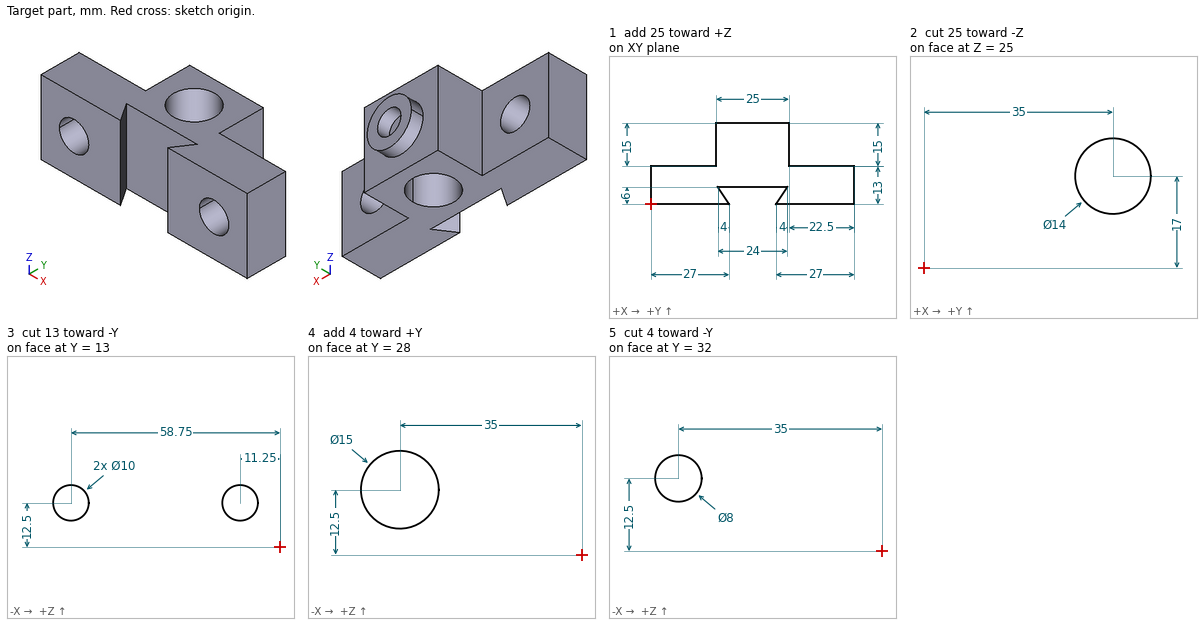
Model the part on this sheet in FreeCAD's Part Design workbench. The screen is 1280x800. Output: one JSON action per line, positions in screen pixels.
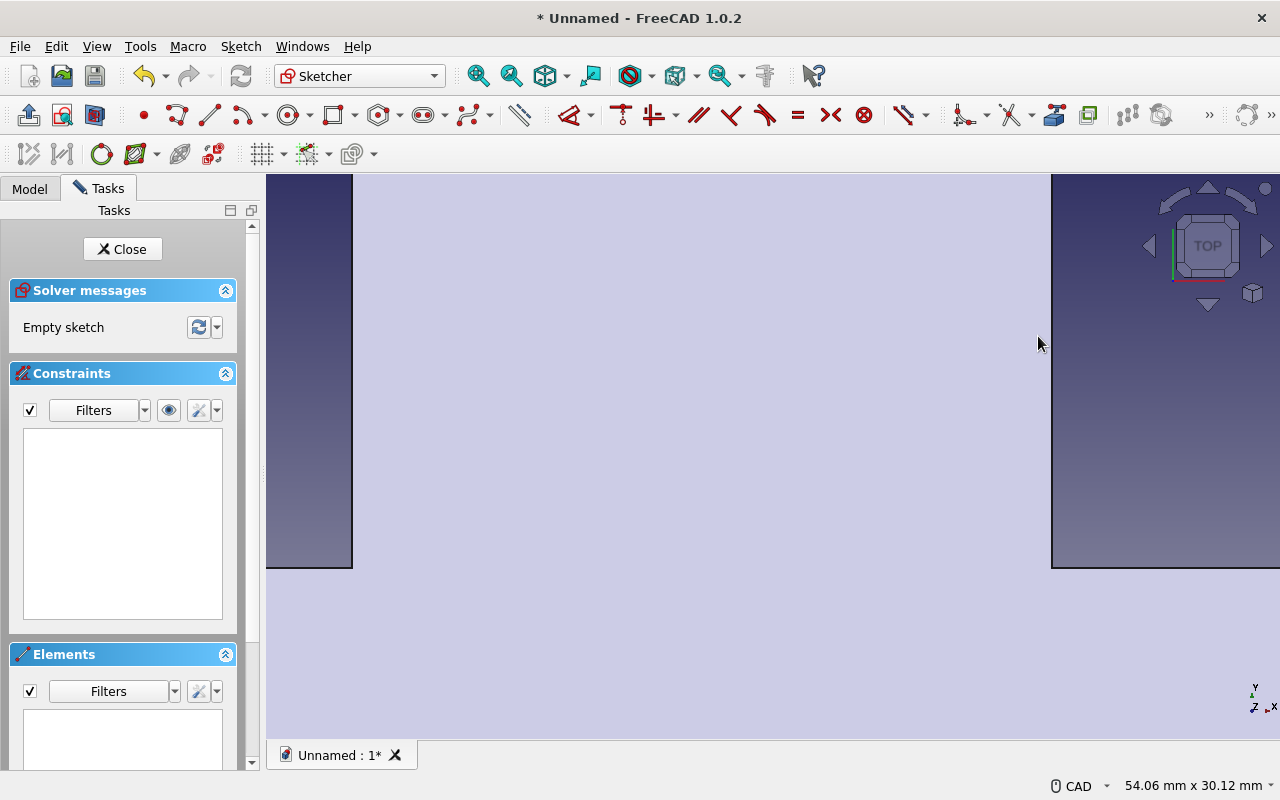
{"action": "left_click", "coordinate": [288, 116]}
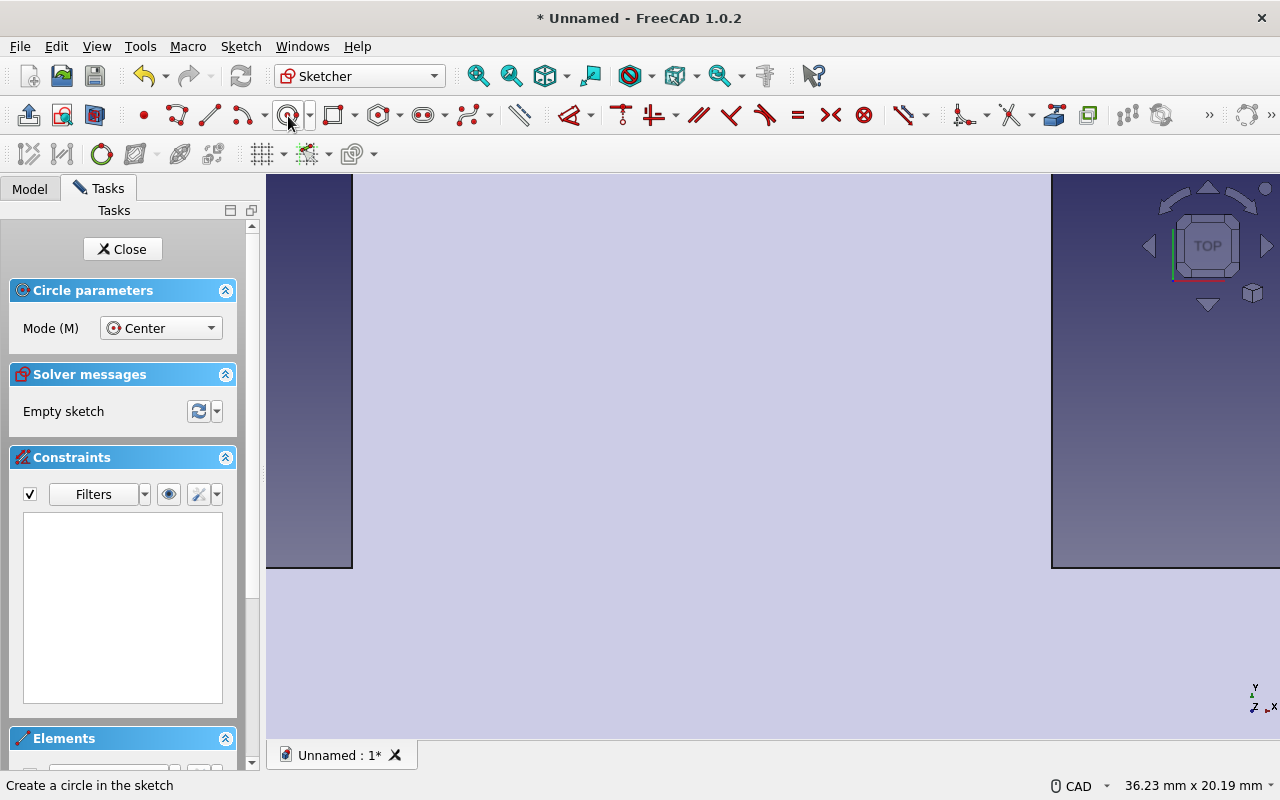
{"action": "left_click", "coordinate": [702, 456]}
{"action": "mouse_move", "coordinate": [840, 317]}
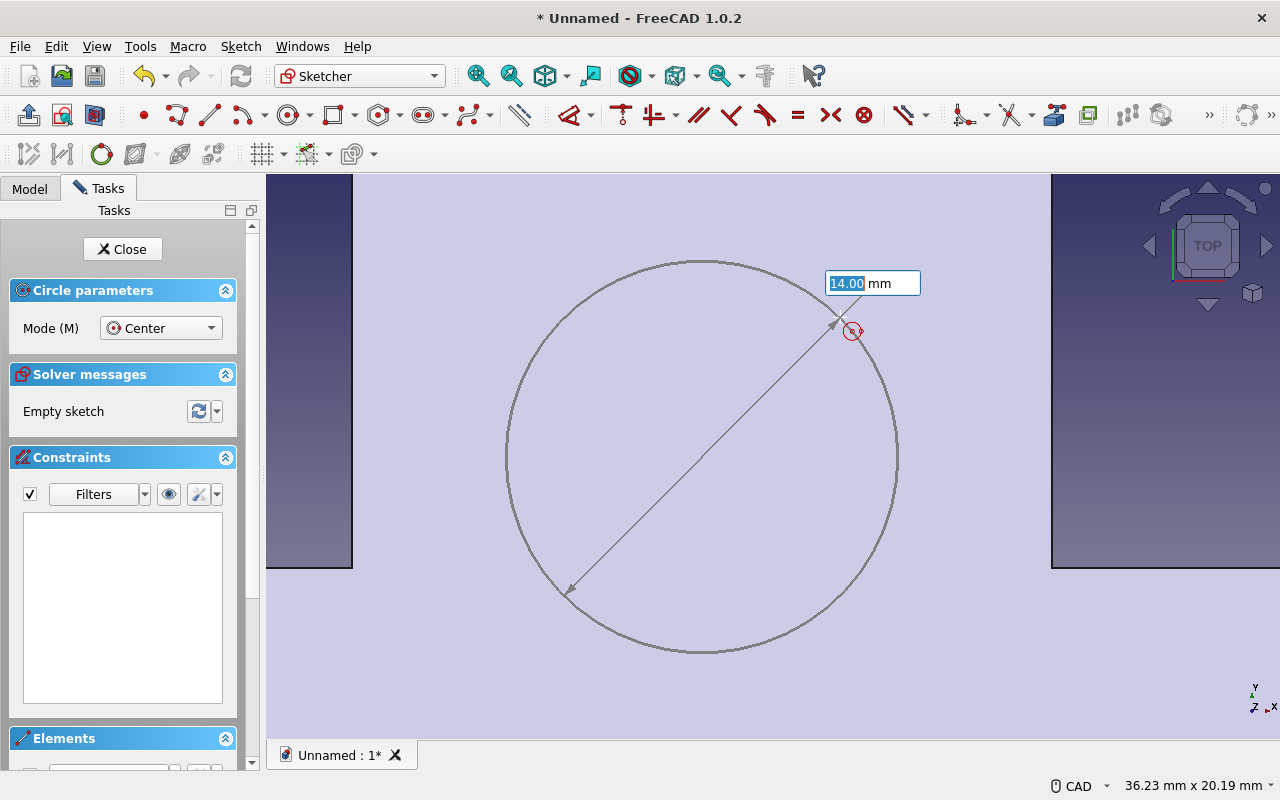
{"action": "type", "text": "14"}
{"action": "key", "text": "Return"}
{"action": "key", "text": "Escape"}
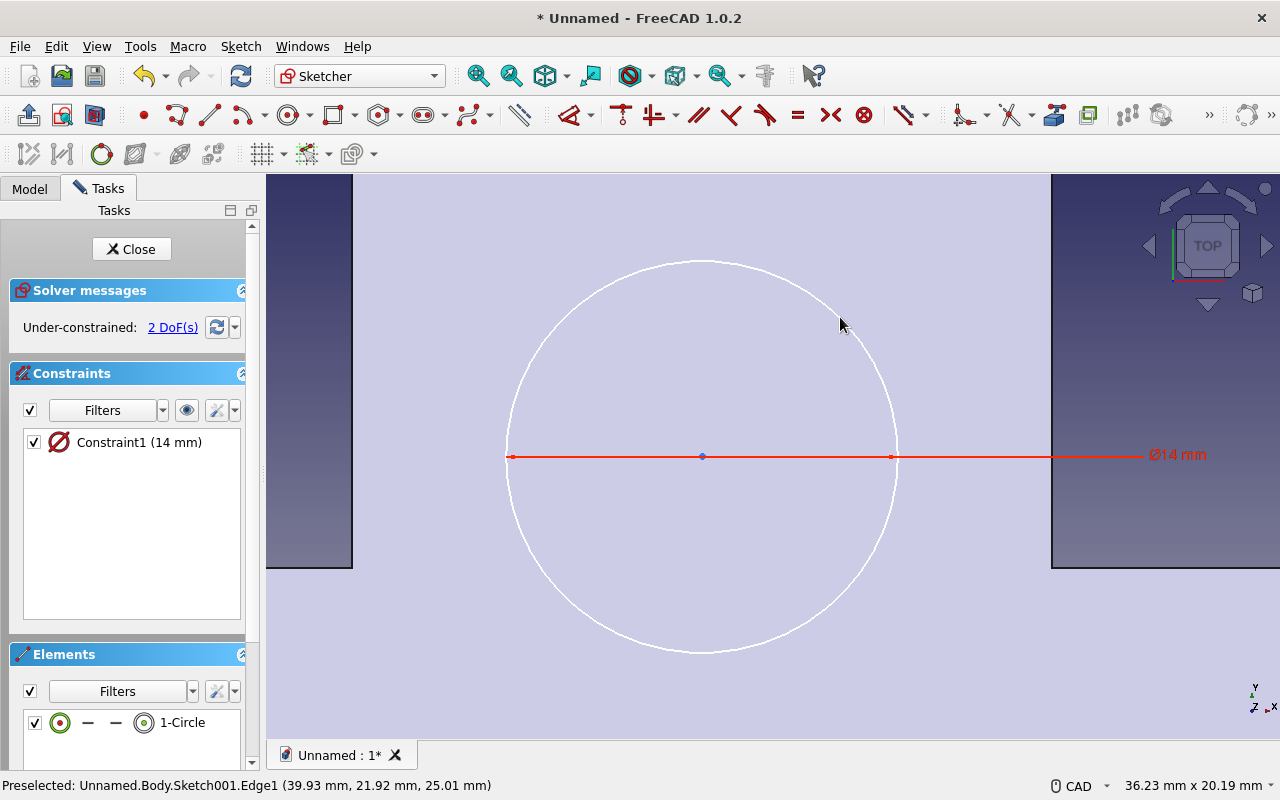
{"action": "left_click", "coordinate": [568, 116]}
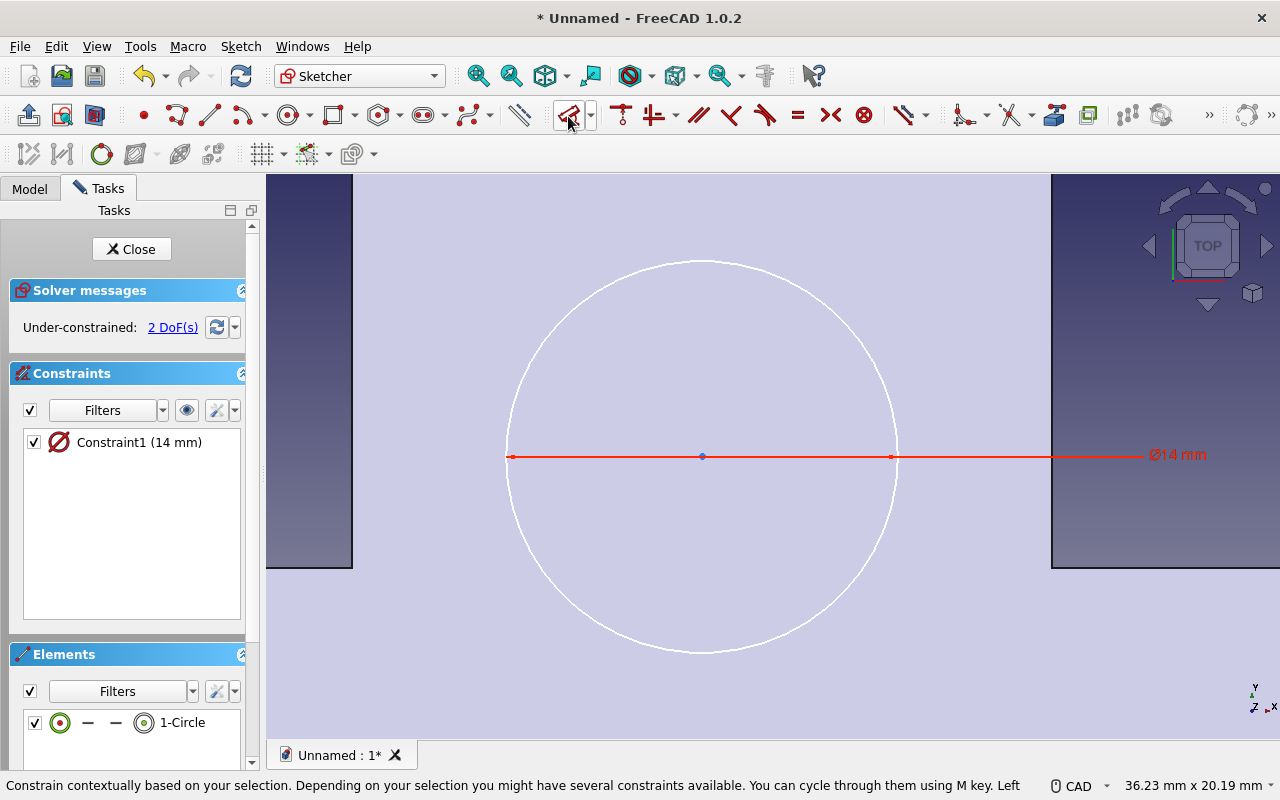
{"action": "left_click", "coordinate": [702, 457]}
{"action": "left_click", "coordinate": [404, 423]}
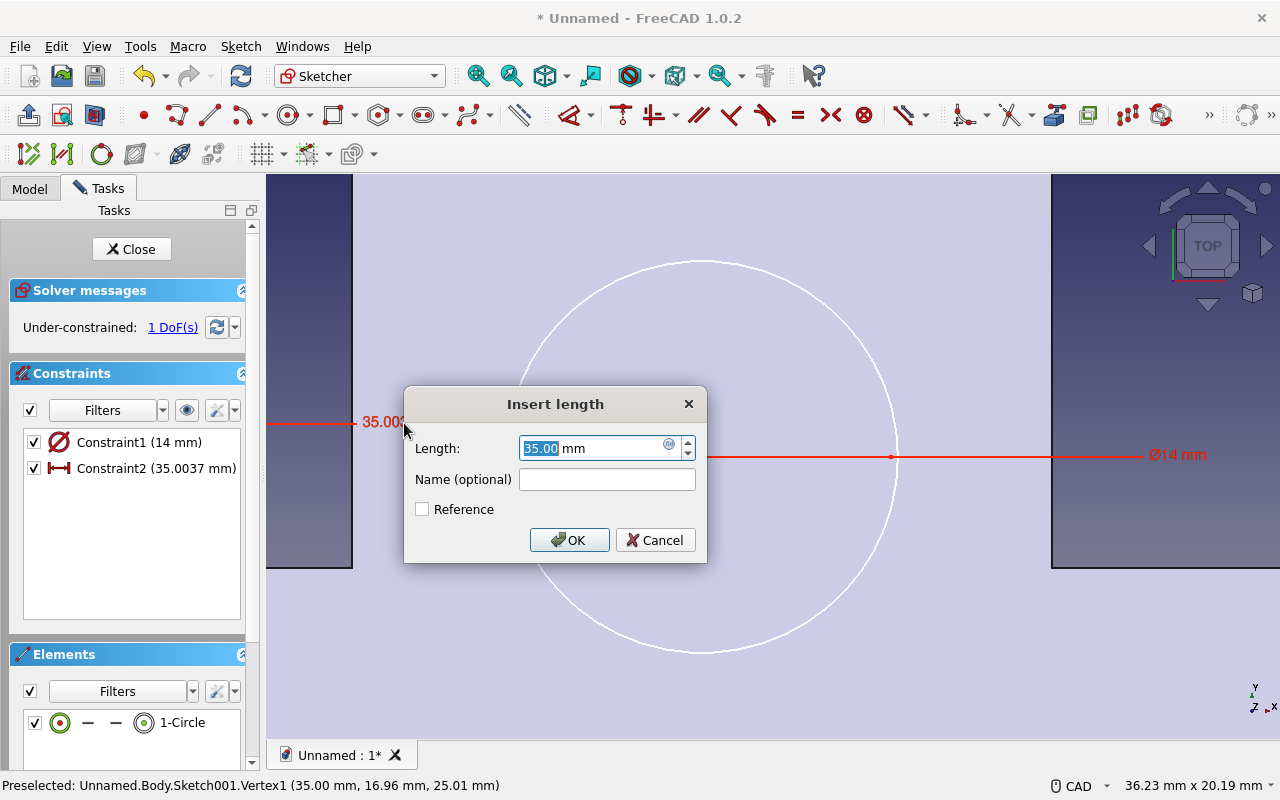
{"action": "type", "text": "35"}
{"action": "key", "text": "Return"}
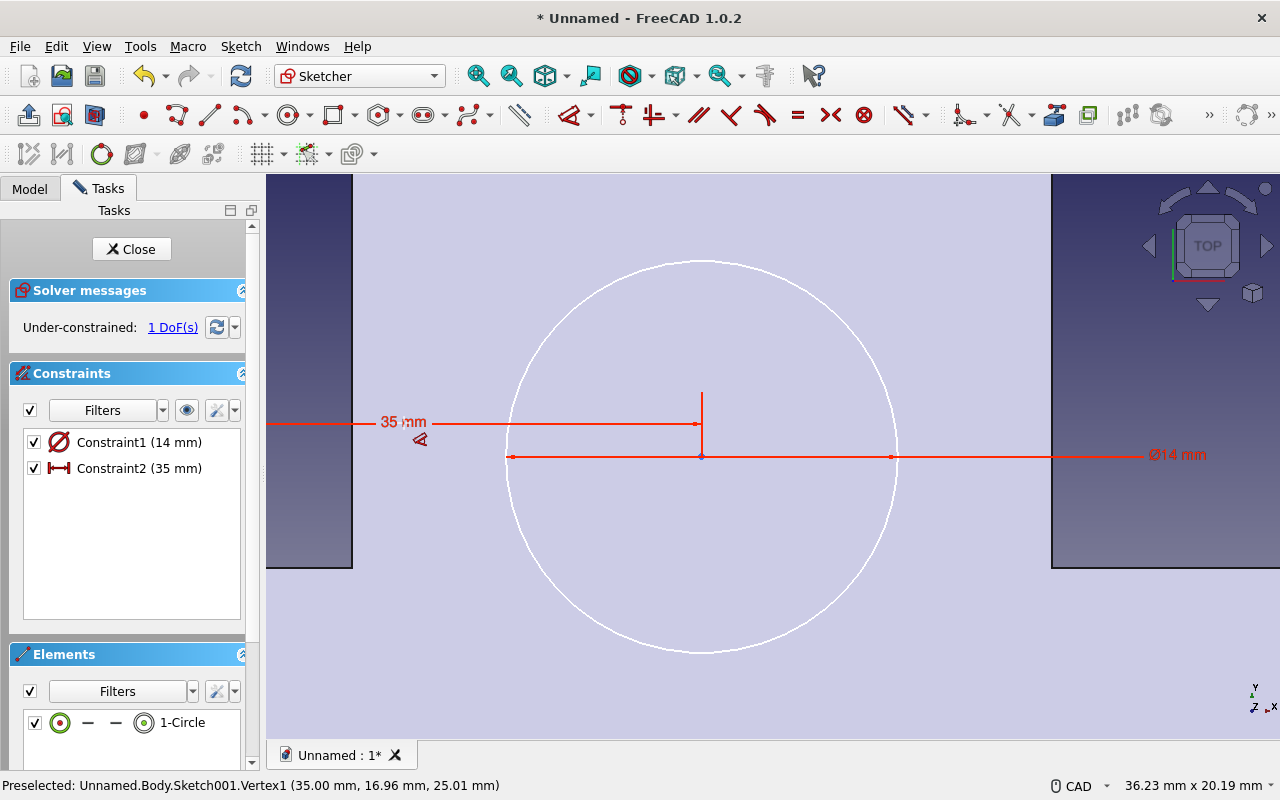
{"action": "left_click", "coordinate": [702, 457]}
{"action": "left_click", "coordinate": [736, 584]}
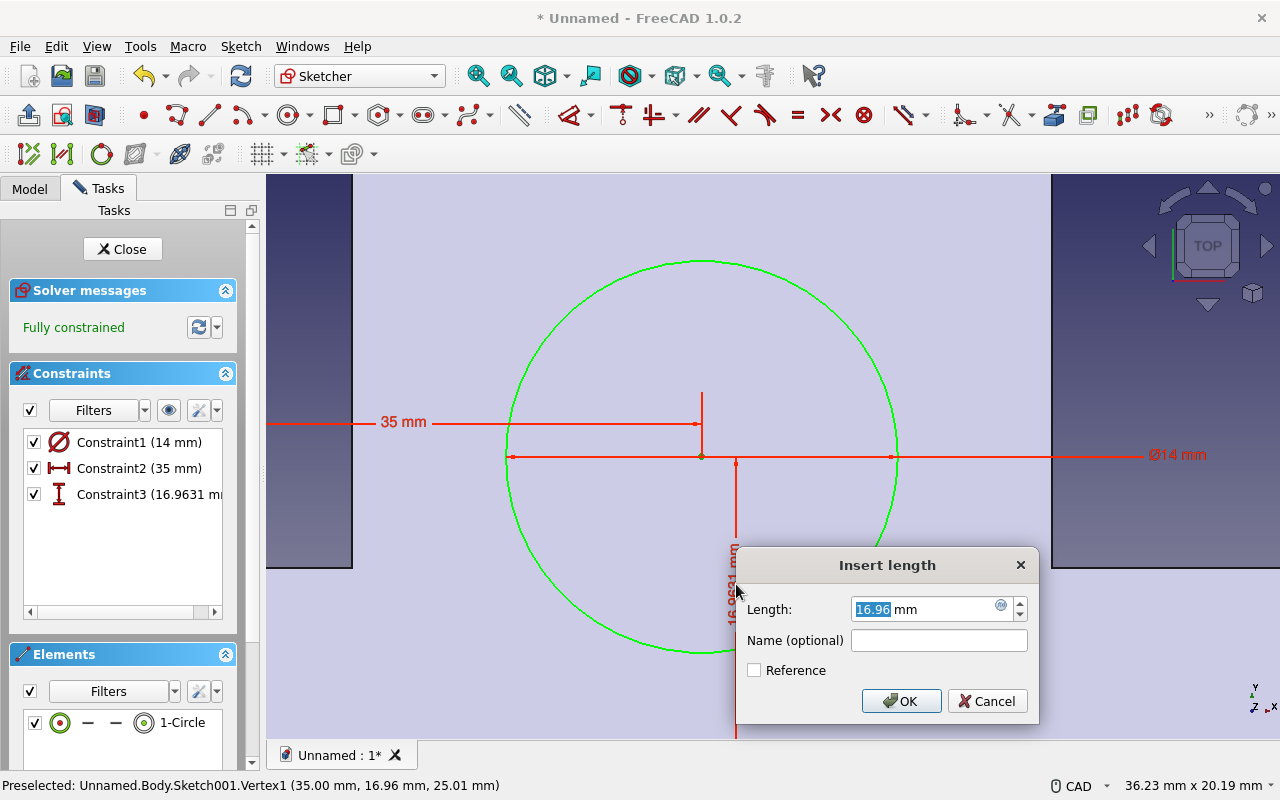
{"action": "type", "text": "17"}
{"action": "key", "text": "Return"}
{"action": "key", "text": "Escape"}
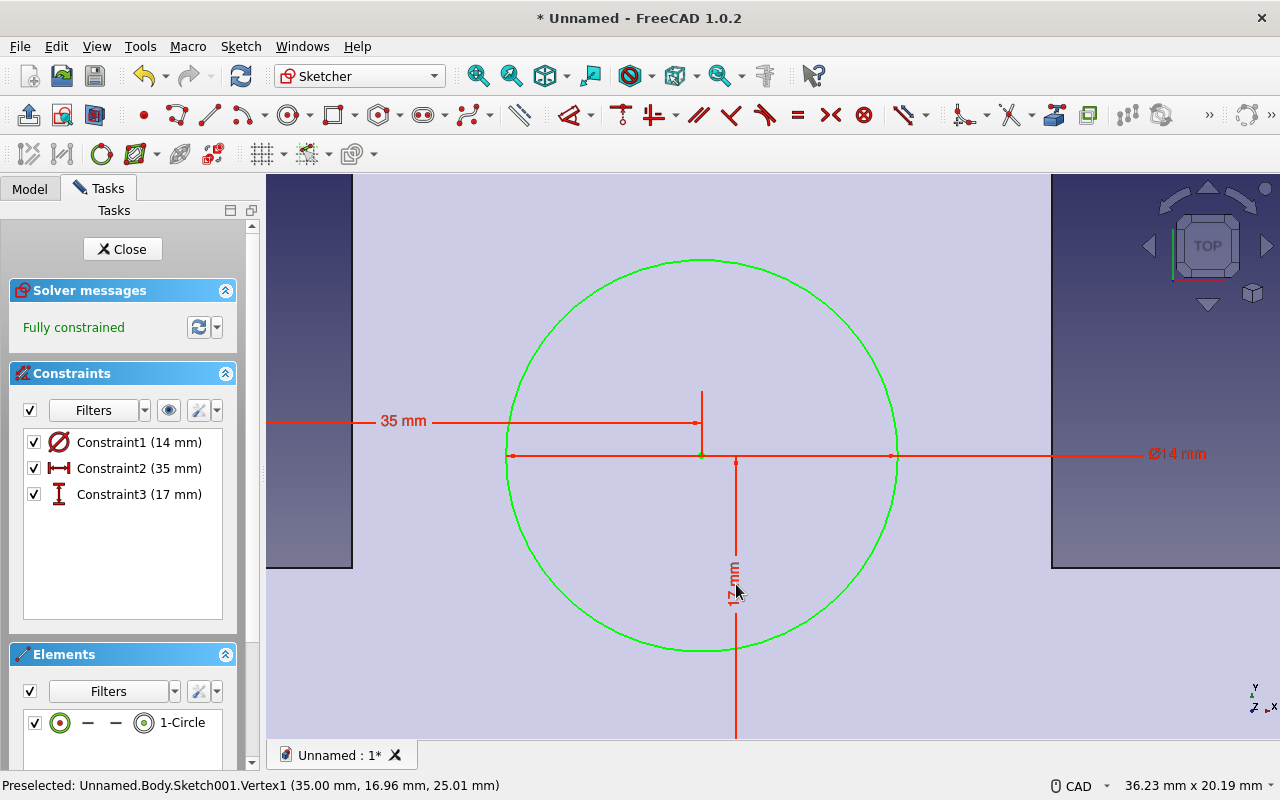
{"action": "left_click", "coordinate": [123, 249]}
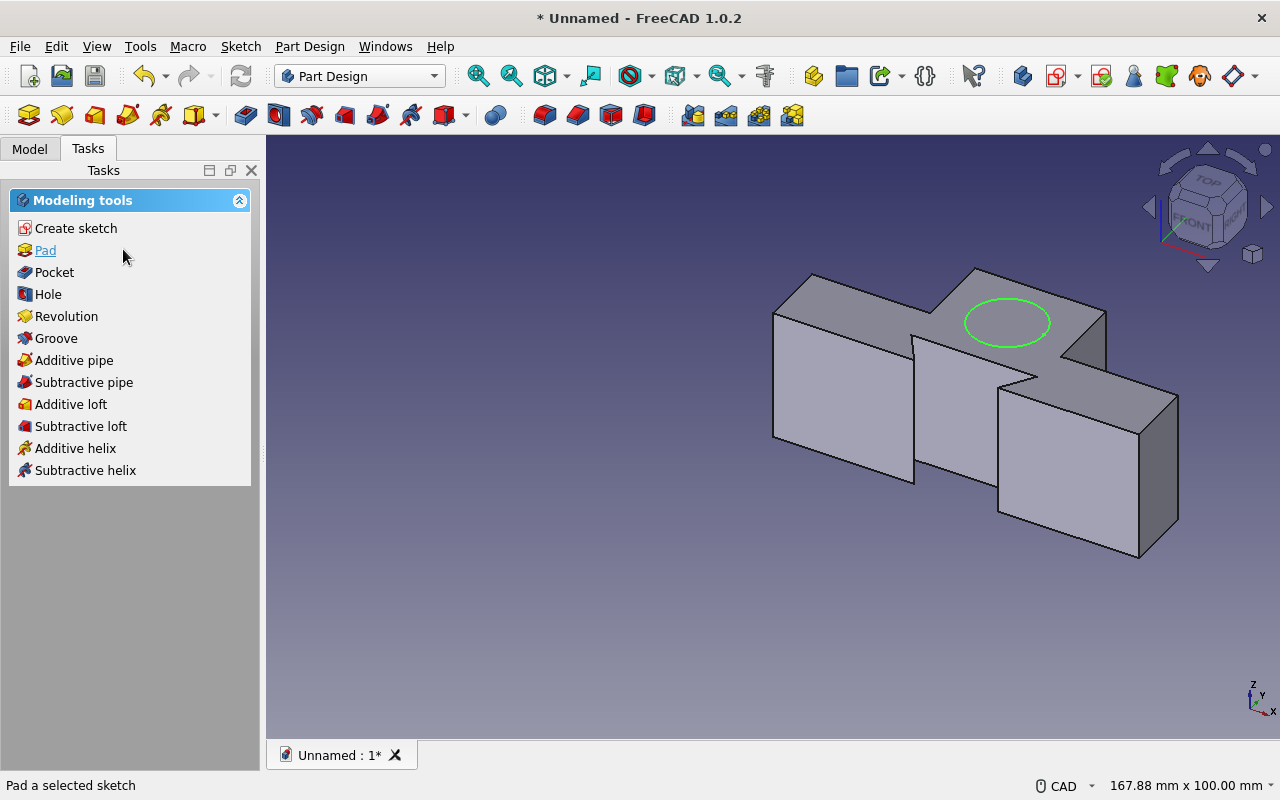
{"action": "left_click", "coordinate": [246, 116]}